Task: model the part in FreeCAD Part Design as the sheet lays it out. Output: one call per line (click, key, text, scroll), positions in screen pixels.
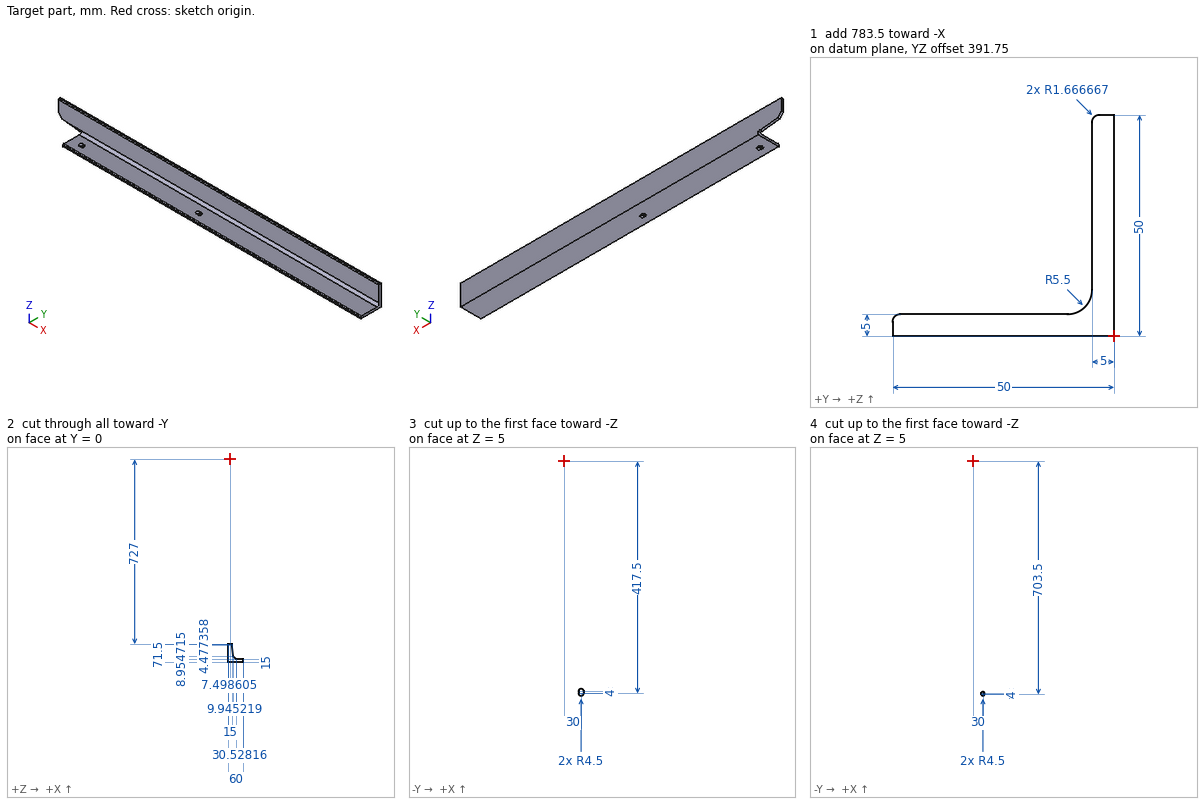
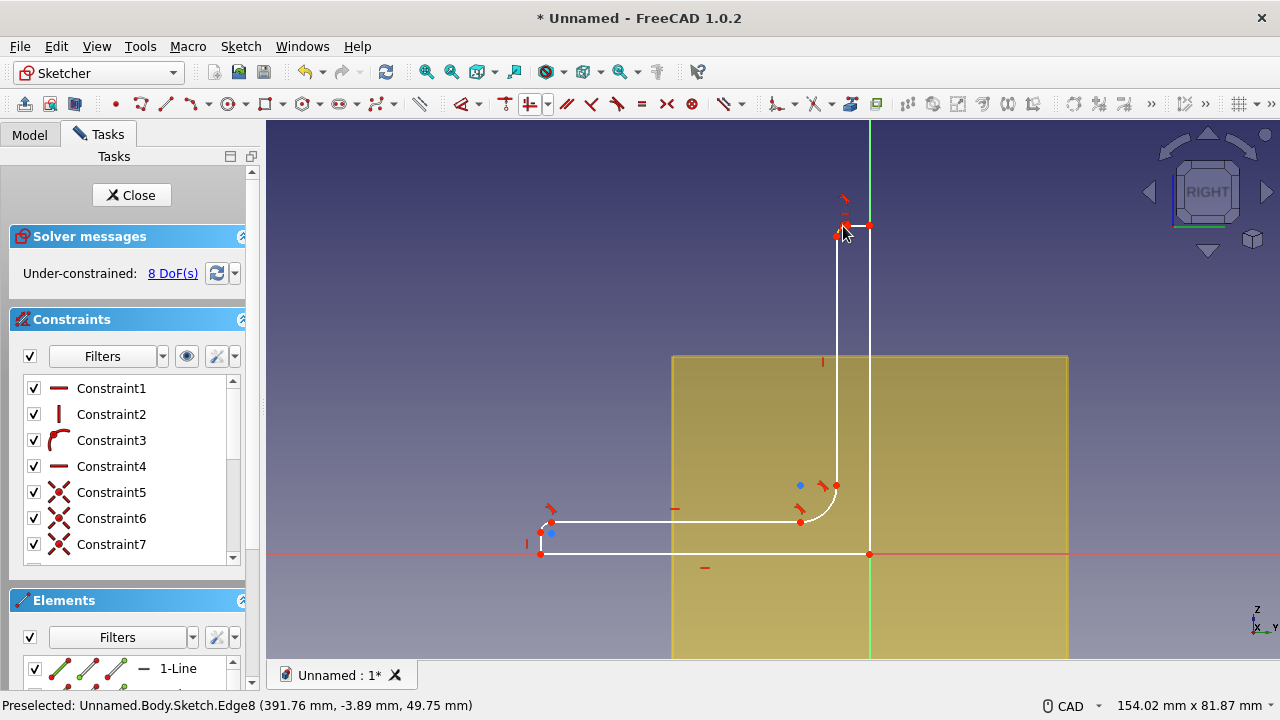
scroll(541, 548, up, 4)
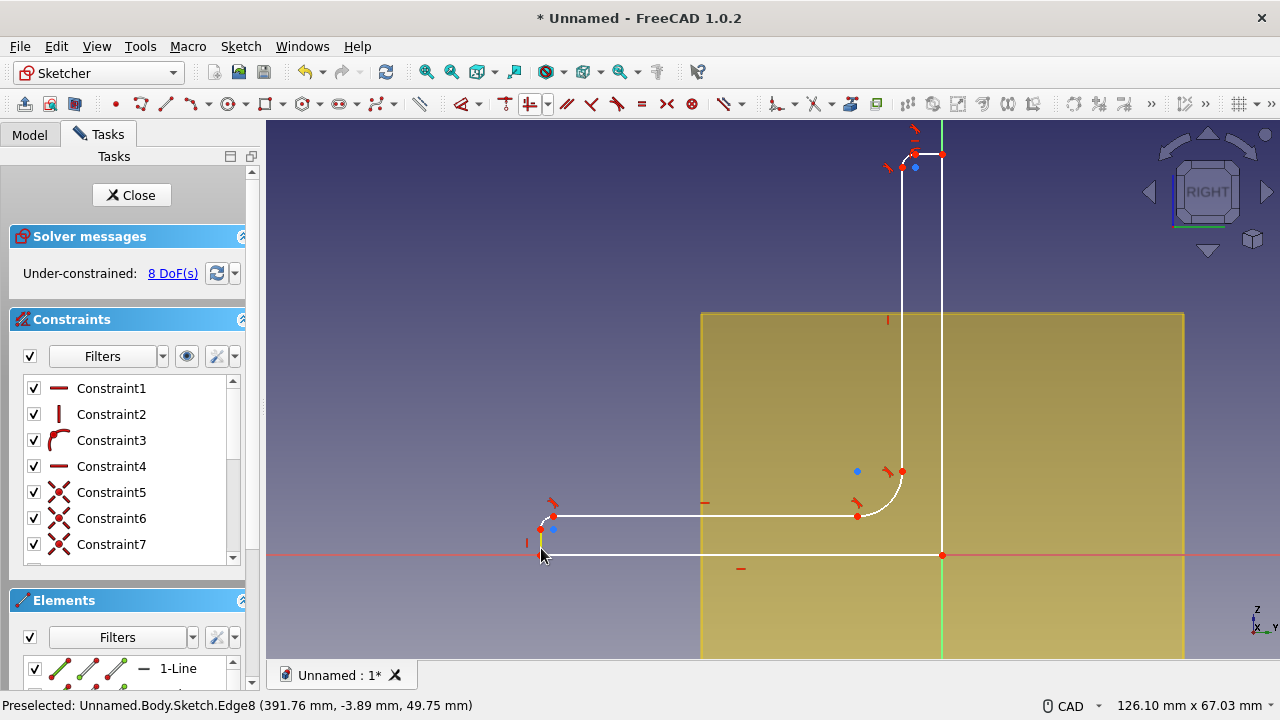
click(540, 546)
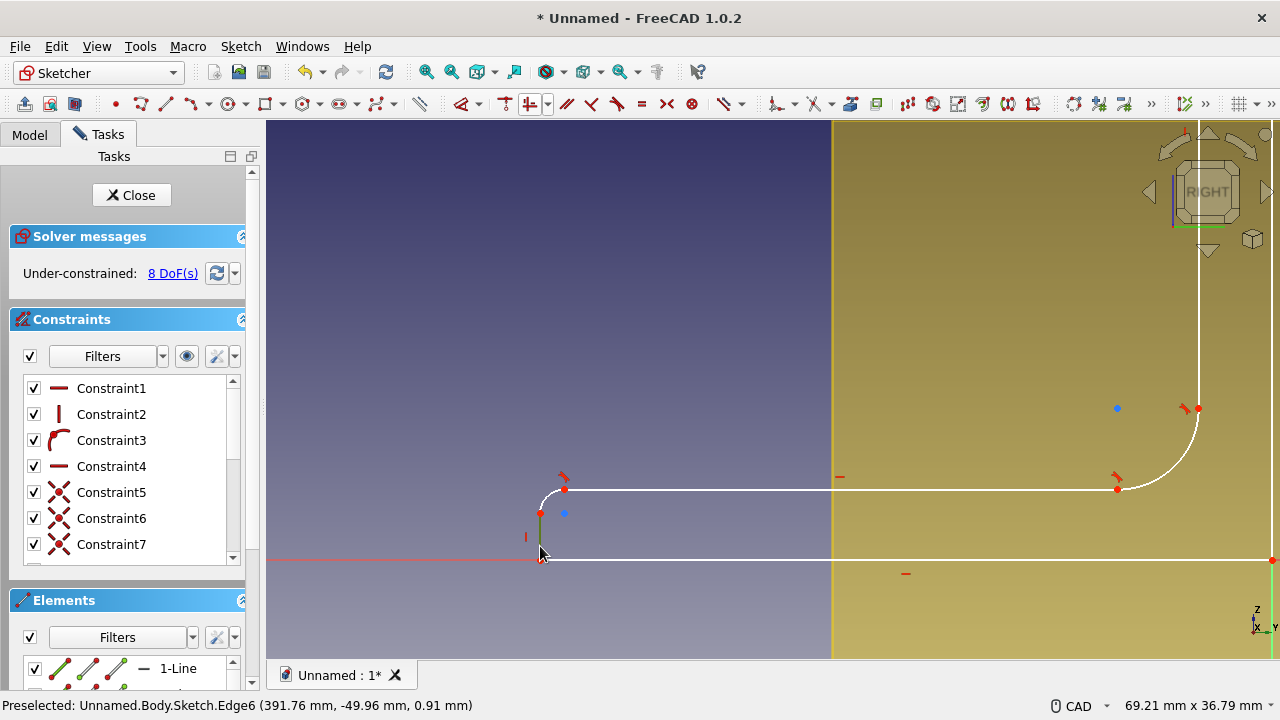
scroll(553, 492, up, 2)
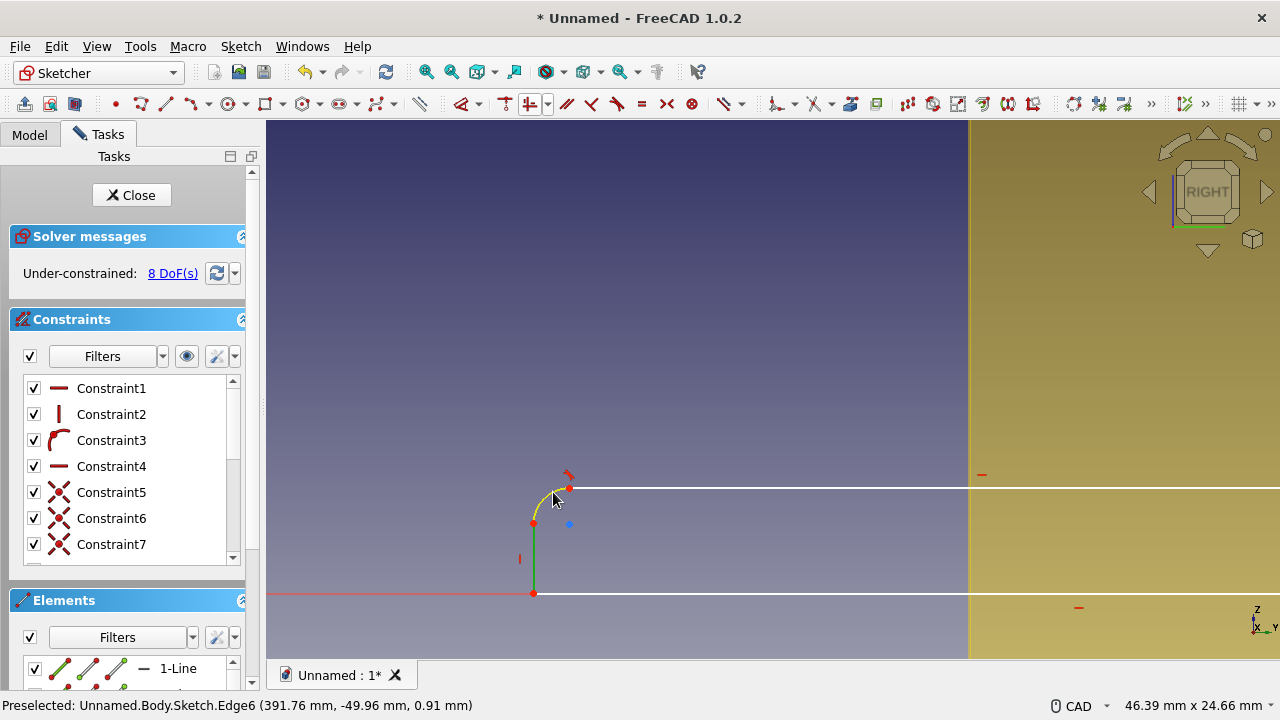
click(553, 492)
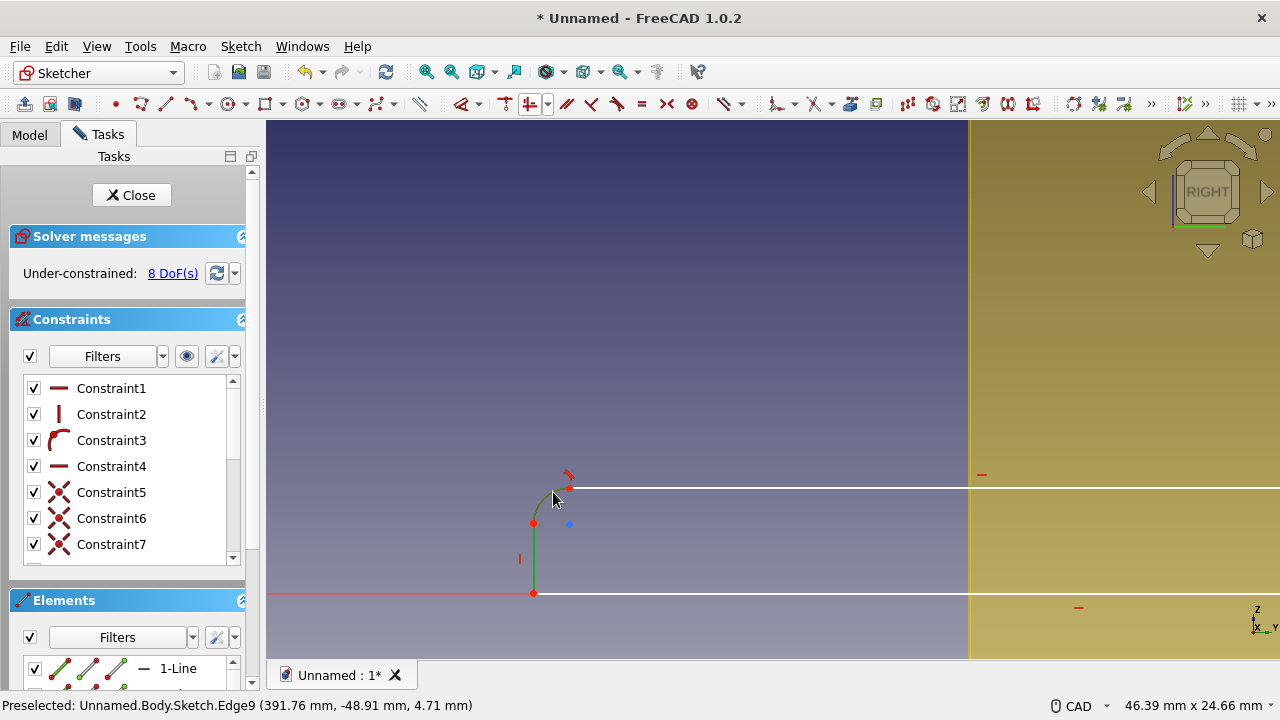
click(617, 104)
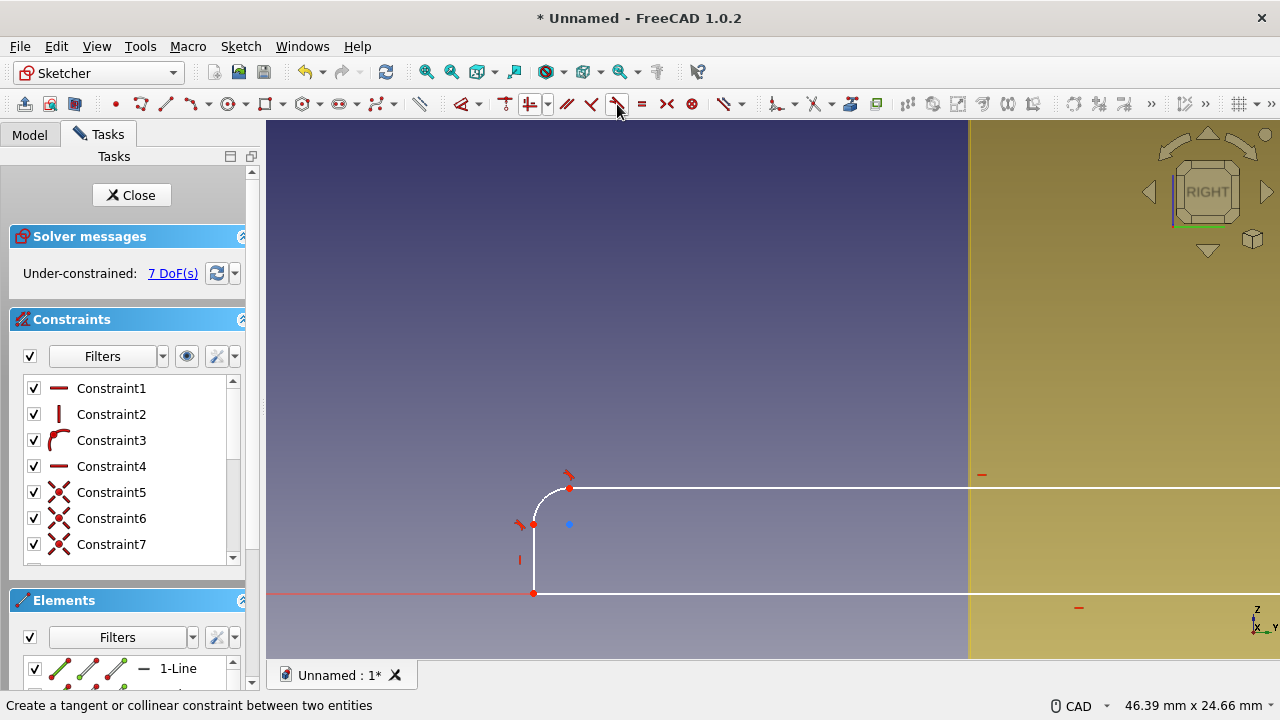
scroll(543, 537, down, 6)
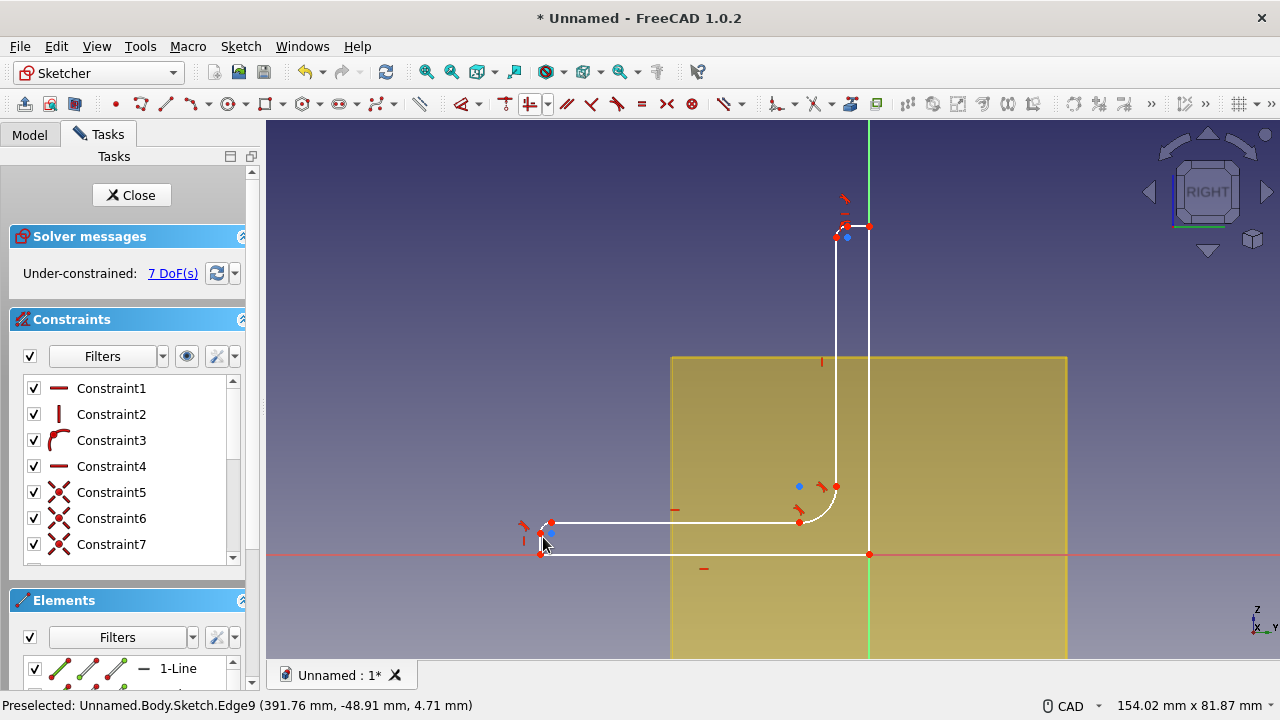
scroll(842, 228, up, 5)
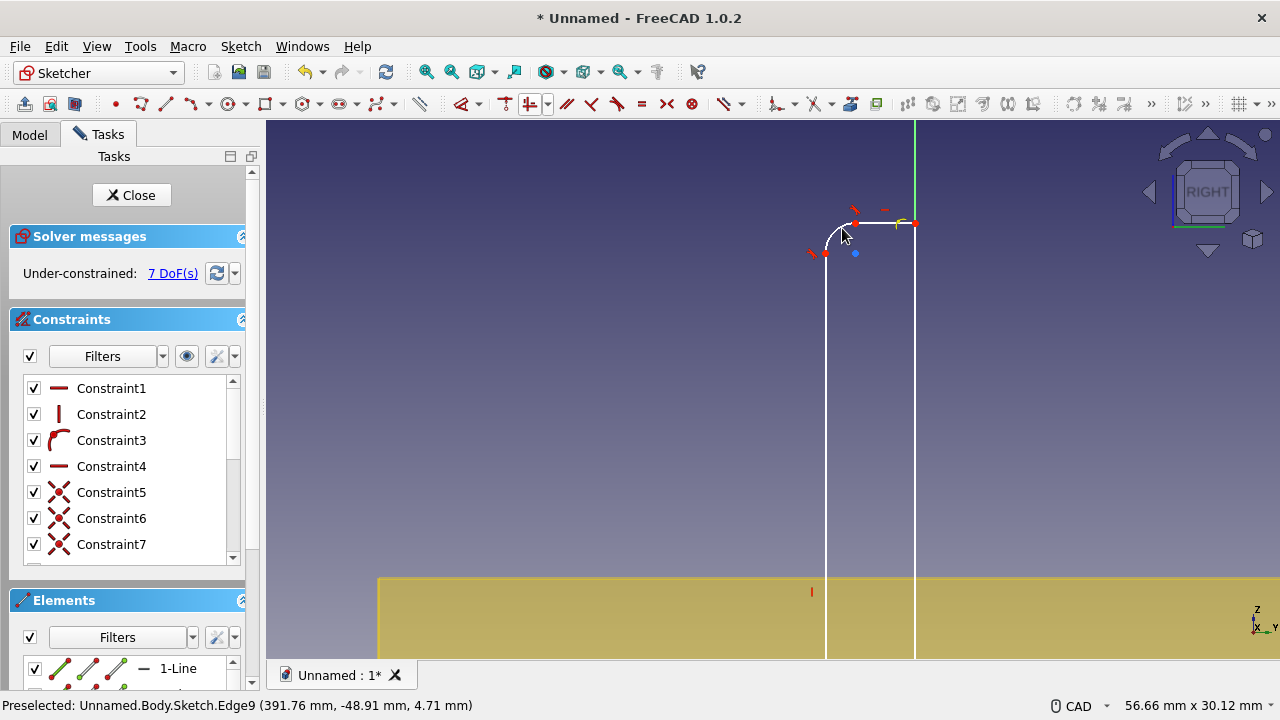
click(842, 226)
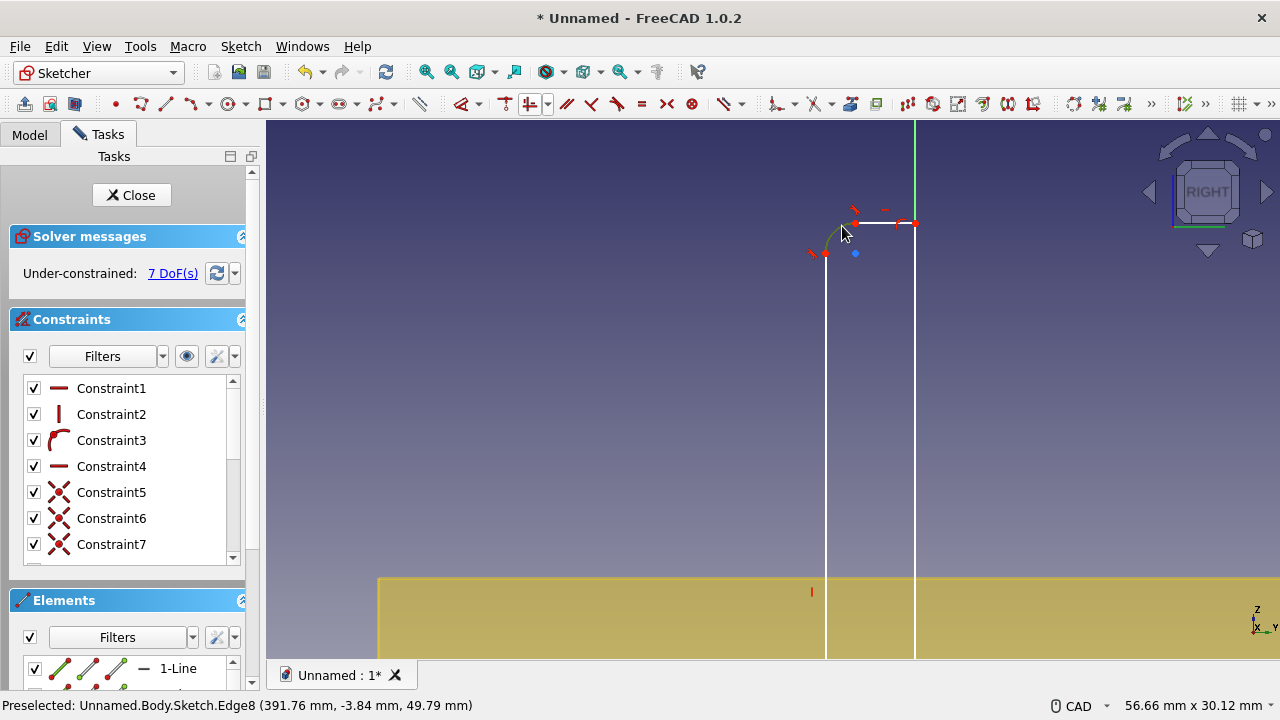
scroll(842, 227, down, 5)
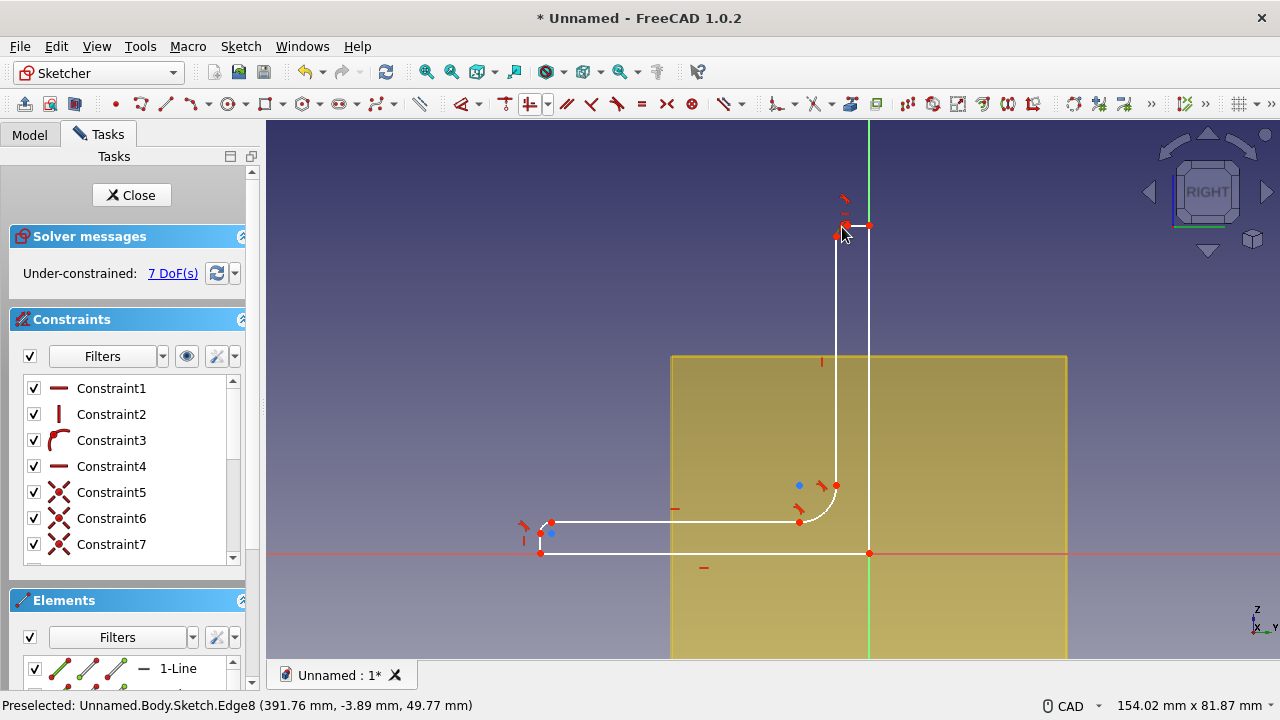
scroll(546, 523, up, 6)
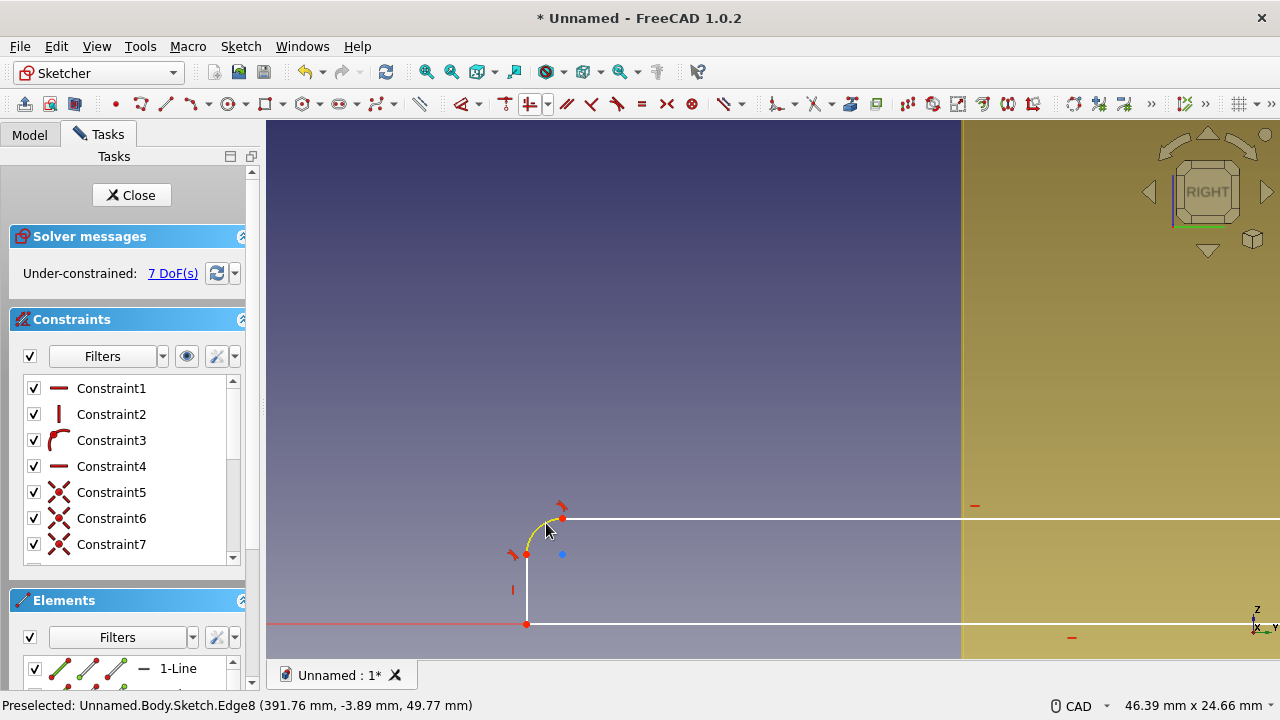
click(546, 523)